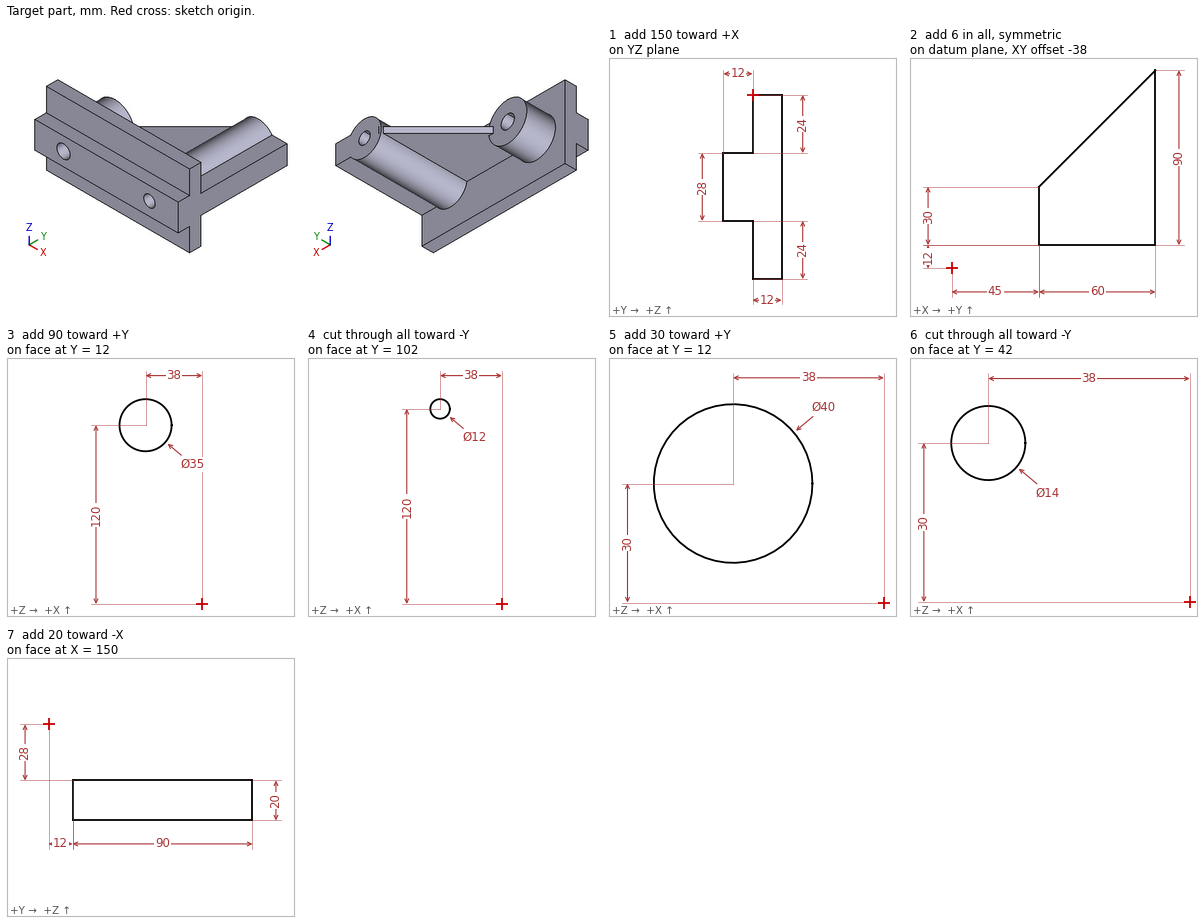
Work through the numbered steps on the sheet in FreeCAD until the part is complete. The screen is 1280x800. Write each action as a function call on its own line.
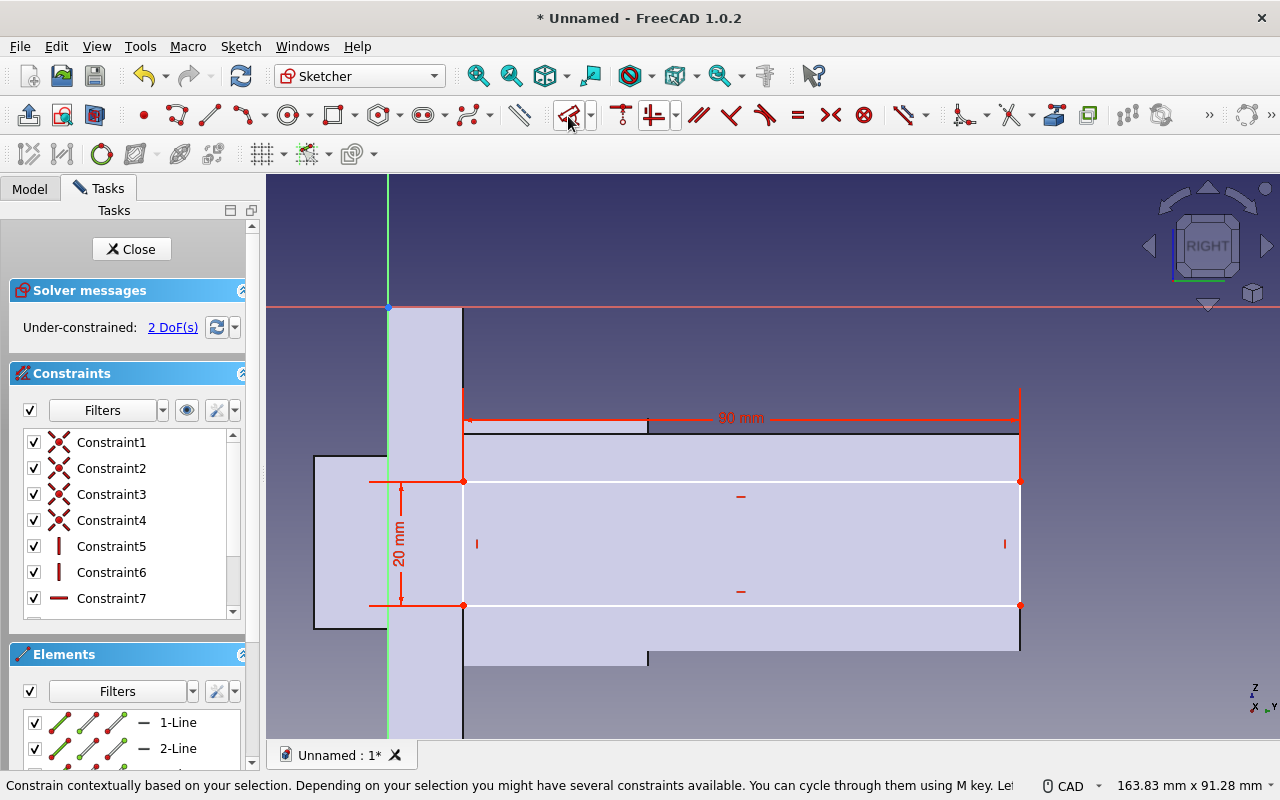
click(463, 482)
click(426, 273)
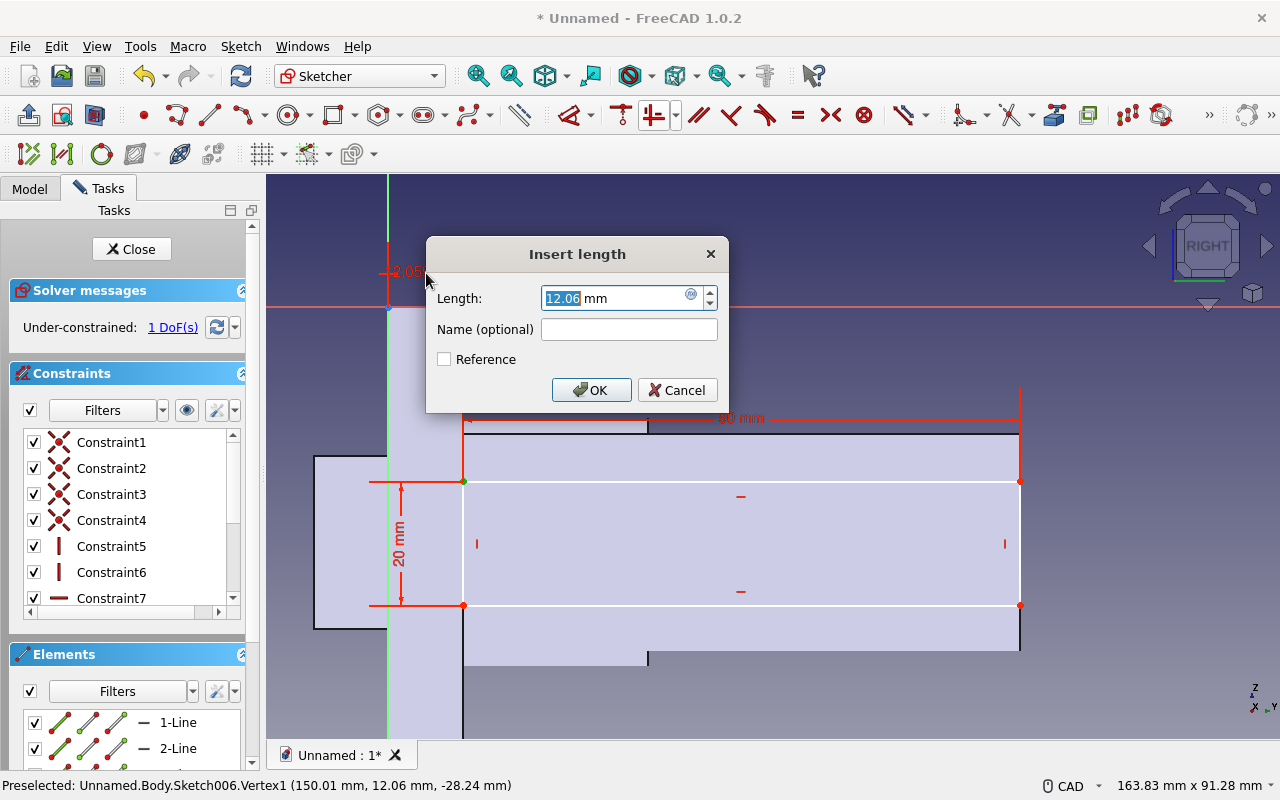
text(12)
key(Return)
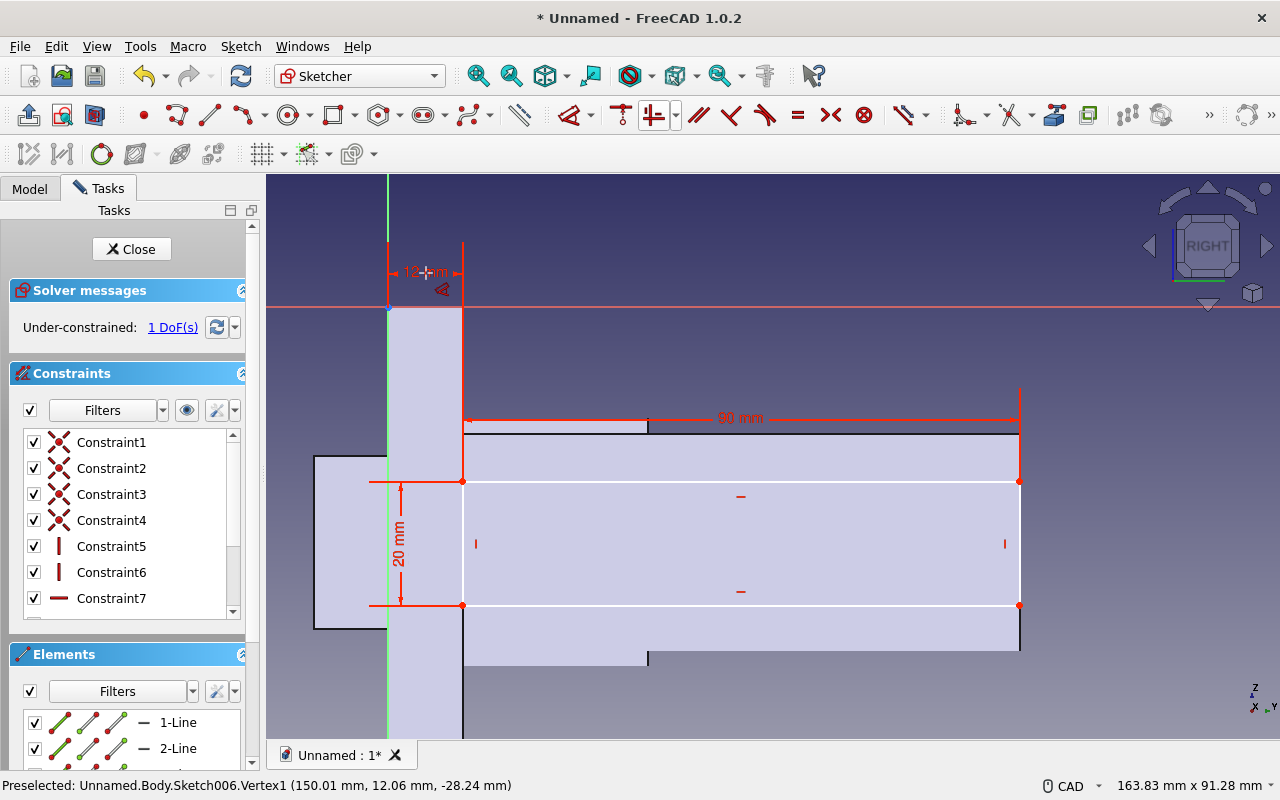
click(463, 482)
click(354, 395)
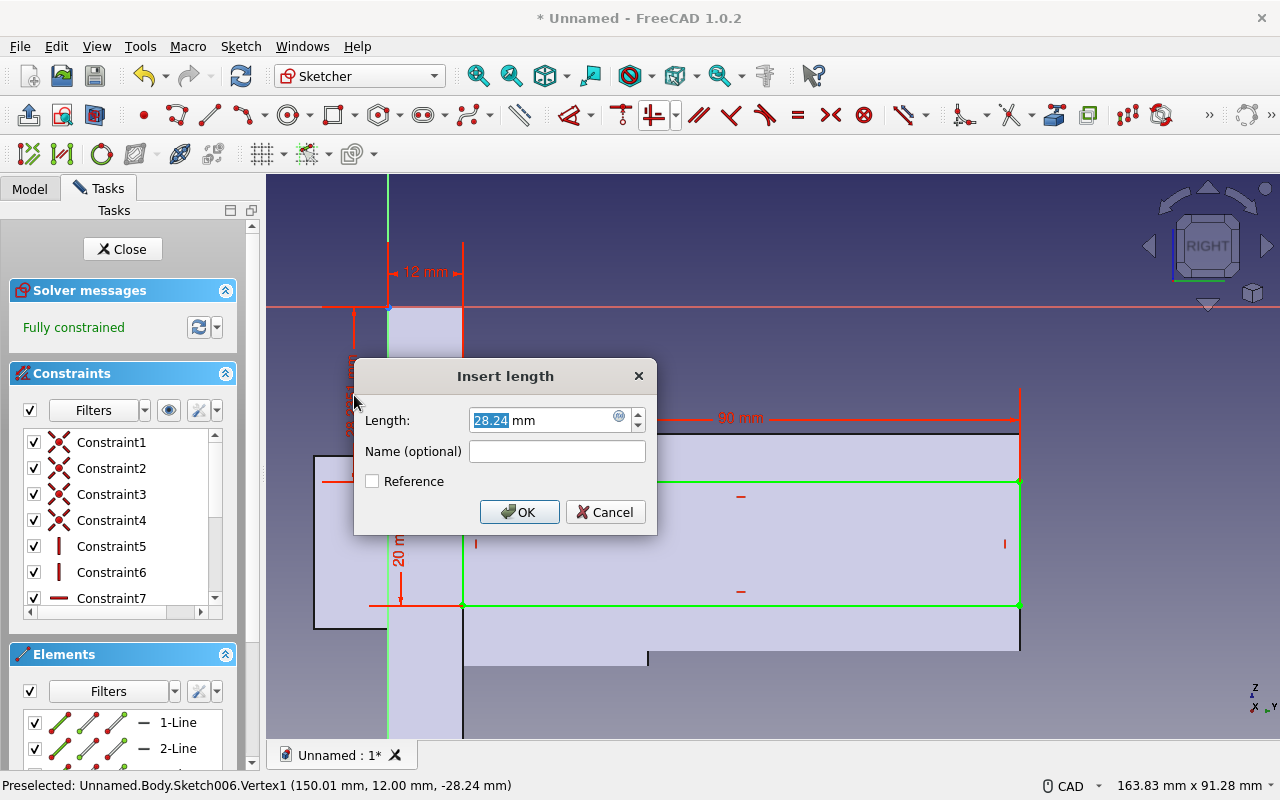
text(28)
key(Return)
key(Escape)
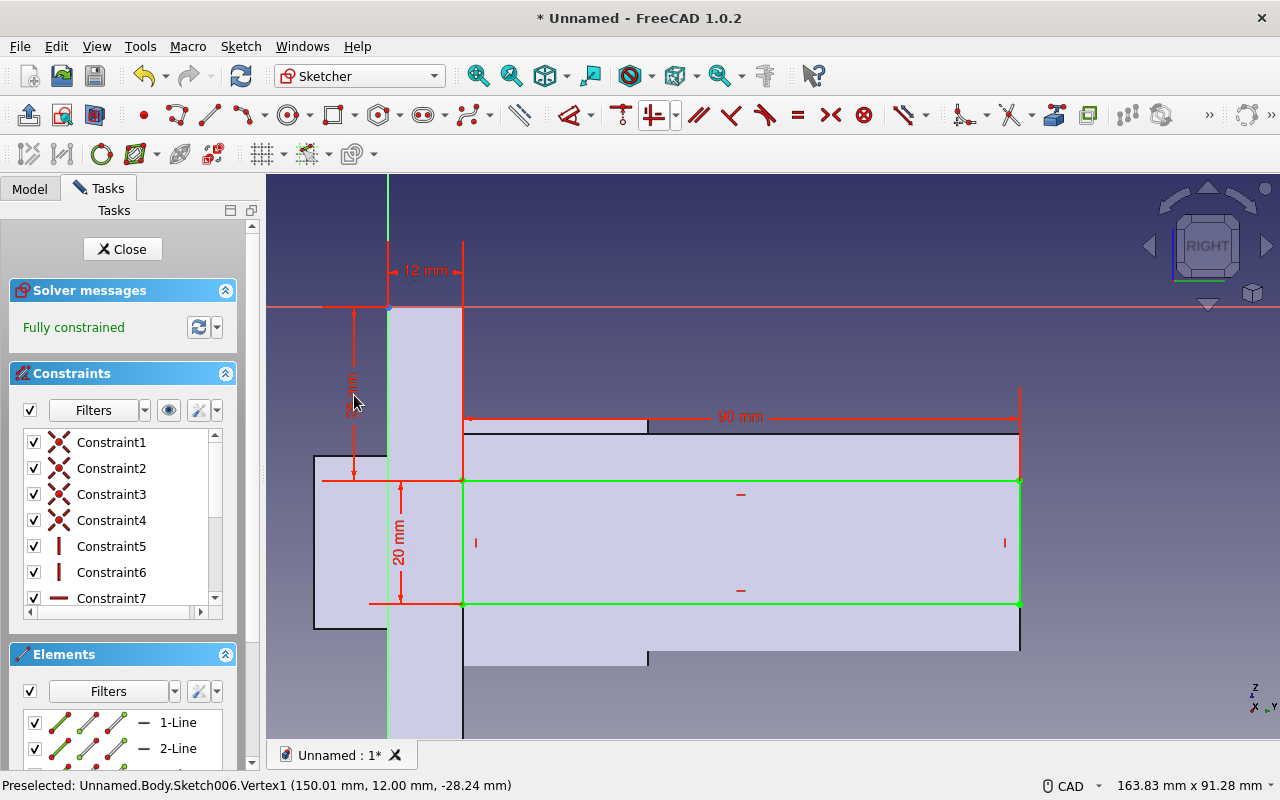
click(123, 249)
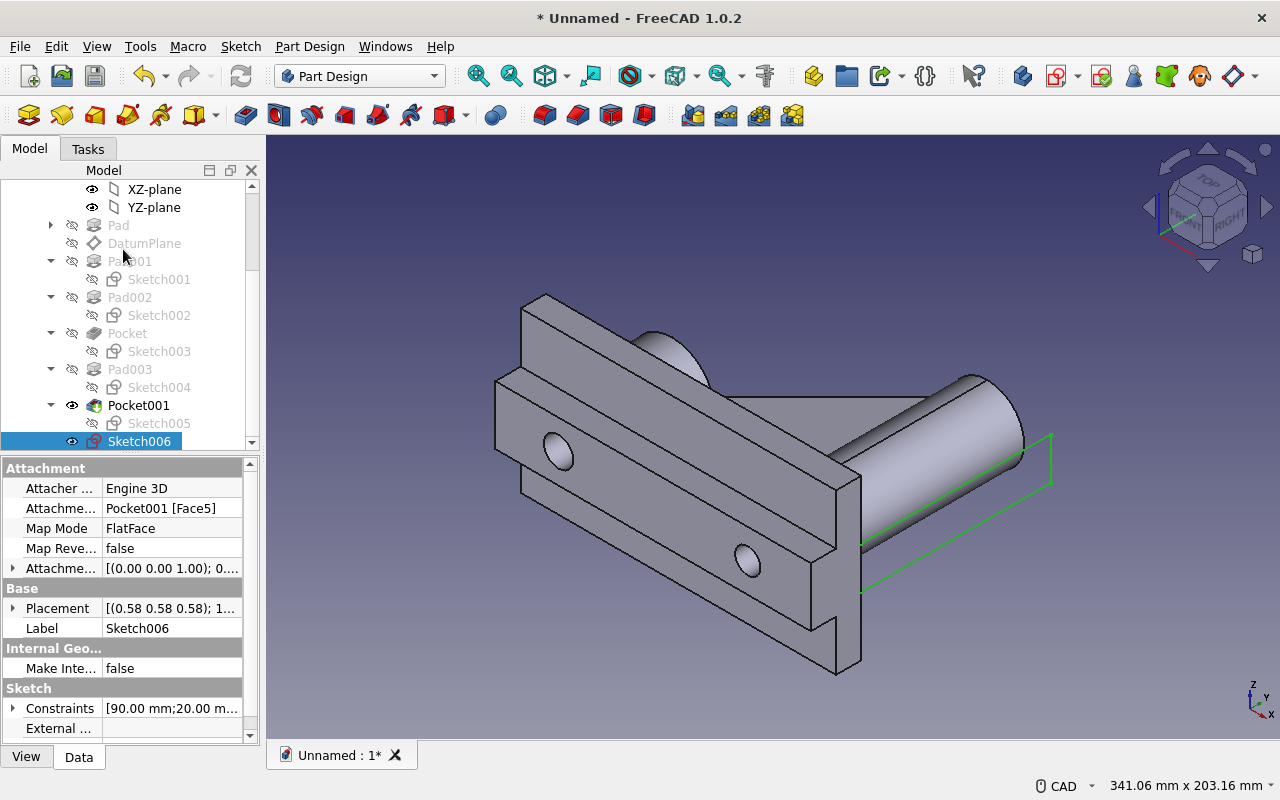
click(29, 116)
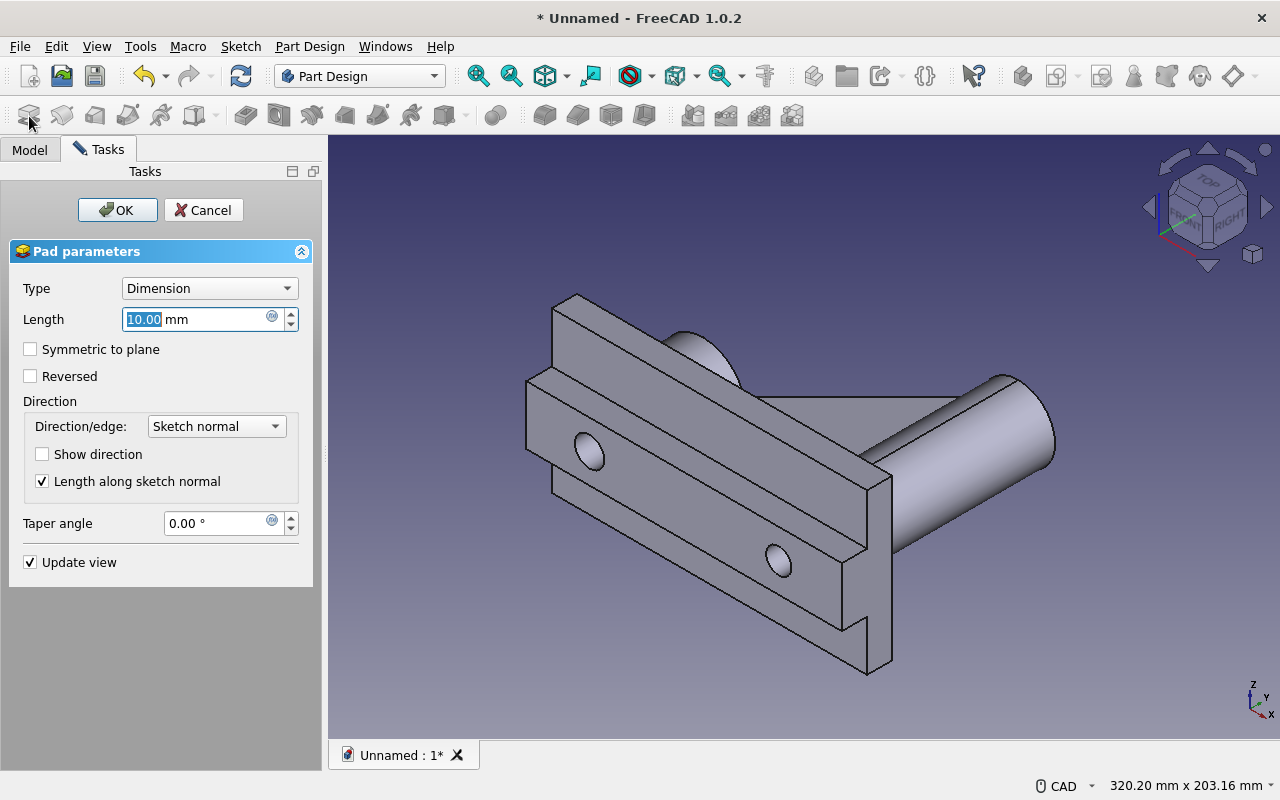
text(20)
key(Tab)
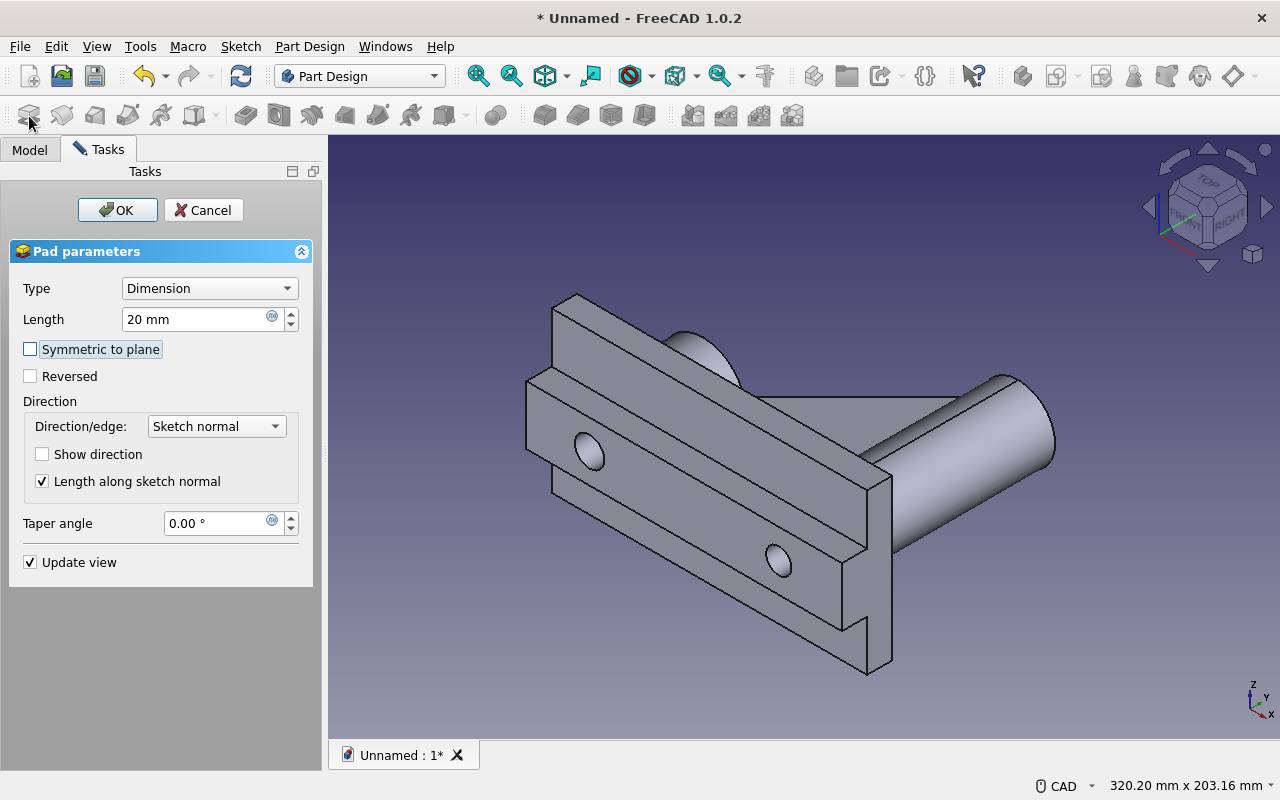
click(31, 376)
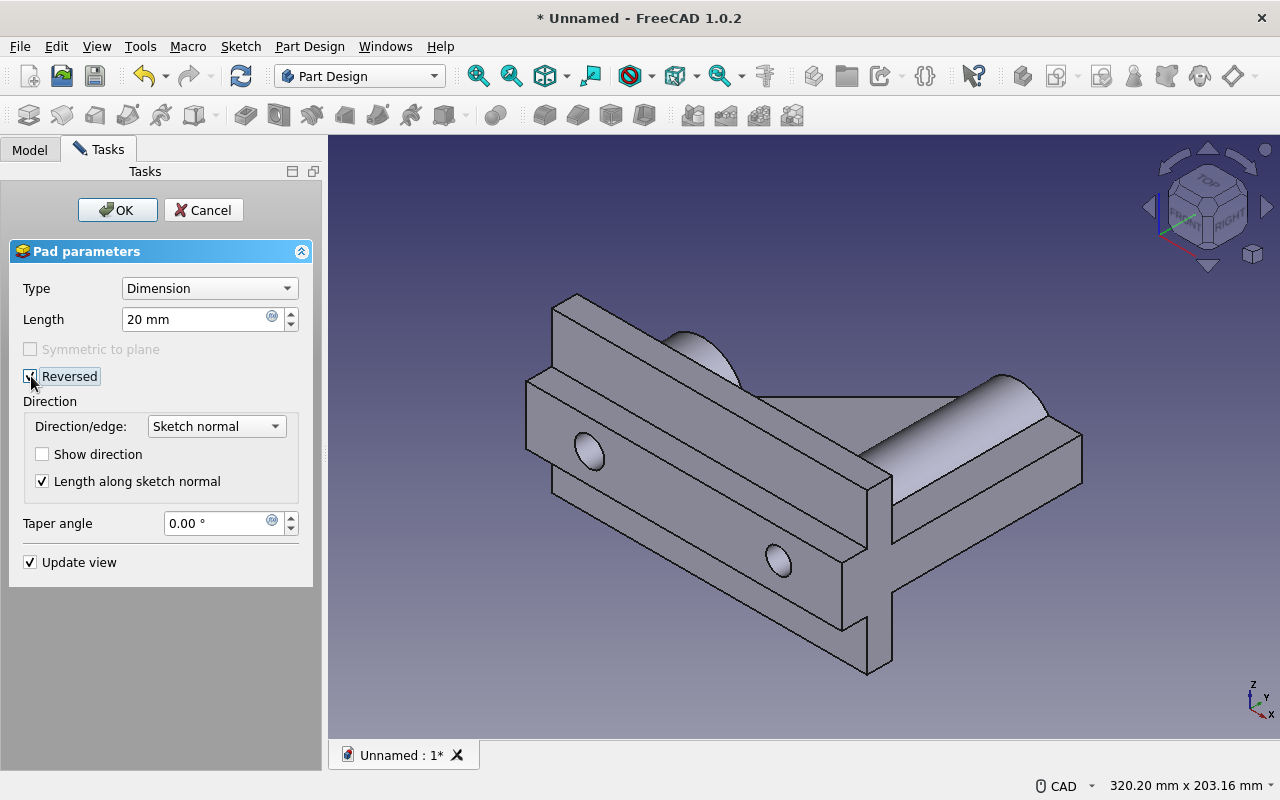
click(118, 210)